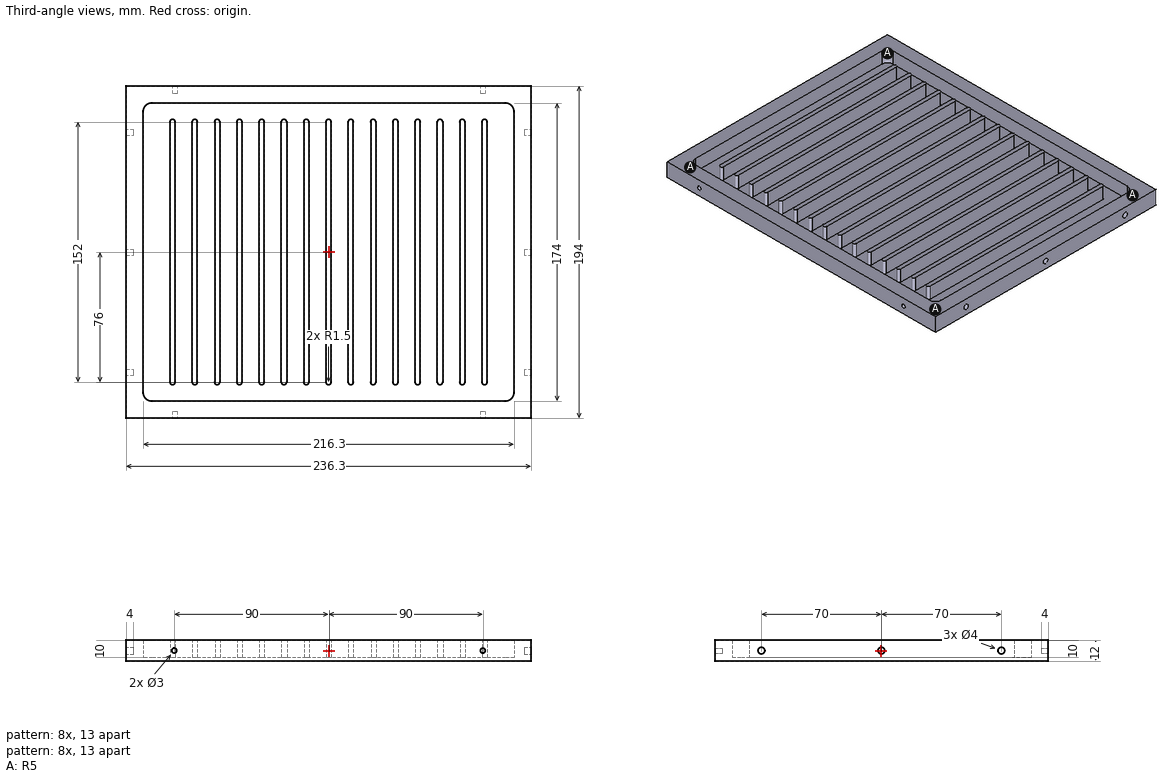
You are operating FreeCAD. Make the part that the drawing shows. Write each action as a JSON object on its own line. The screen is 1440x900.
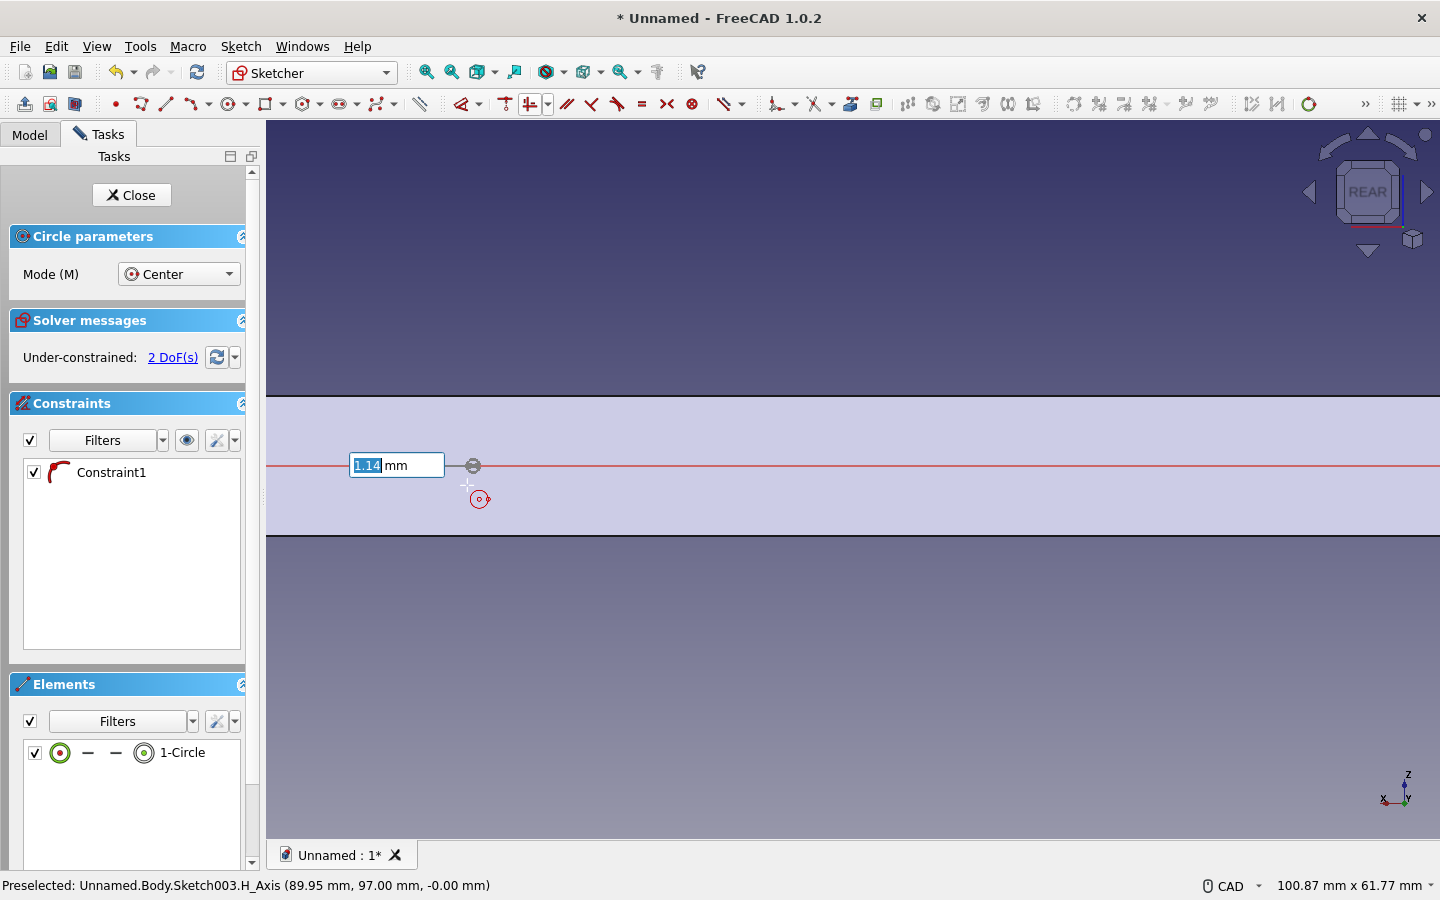
{"action": "left_click", "coordinate": [467, 482]}
{"action": "key", "text": "Escape"}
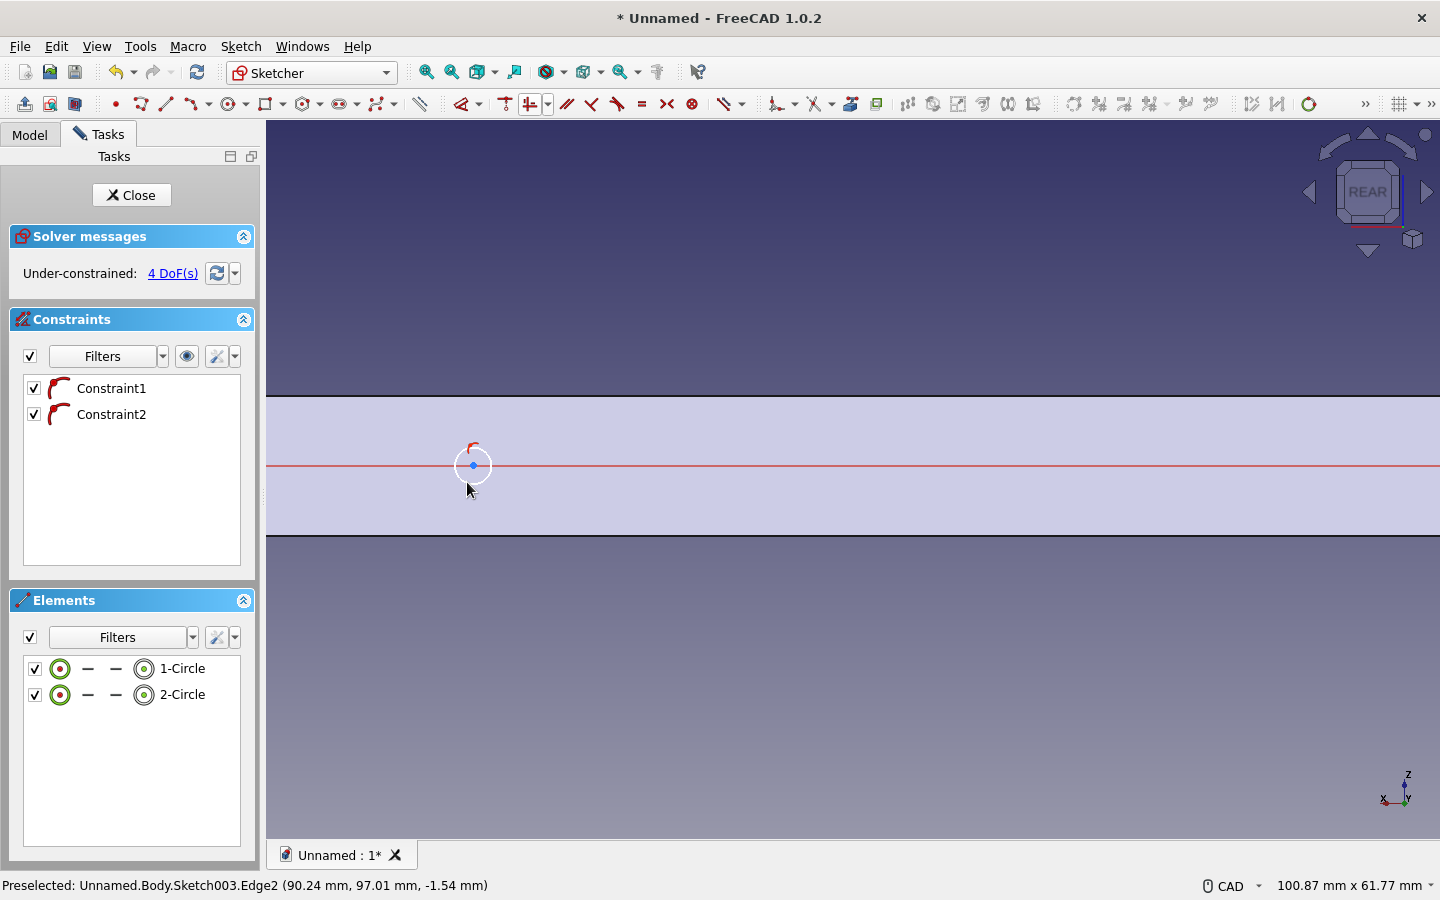
{"action": "scroll", "coordinate": [467, 485], "scroll_direction": "down", "scroll_amount": 6}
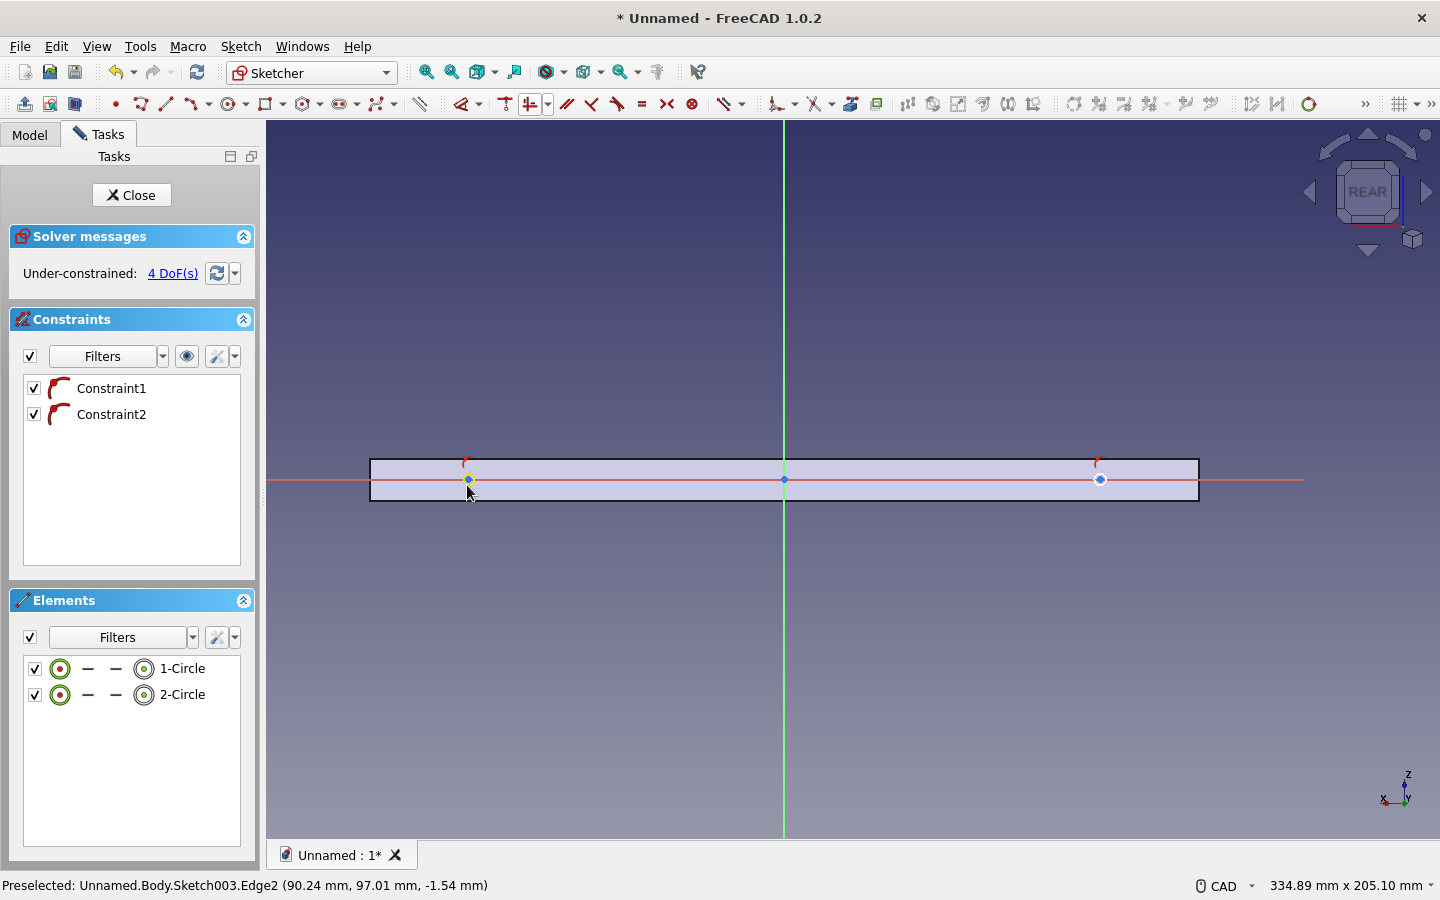
{"action": "scroll", "coordinate": [1104, 476], "scroll_direction": "up", "scroll_amount": 7}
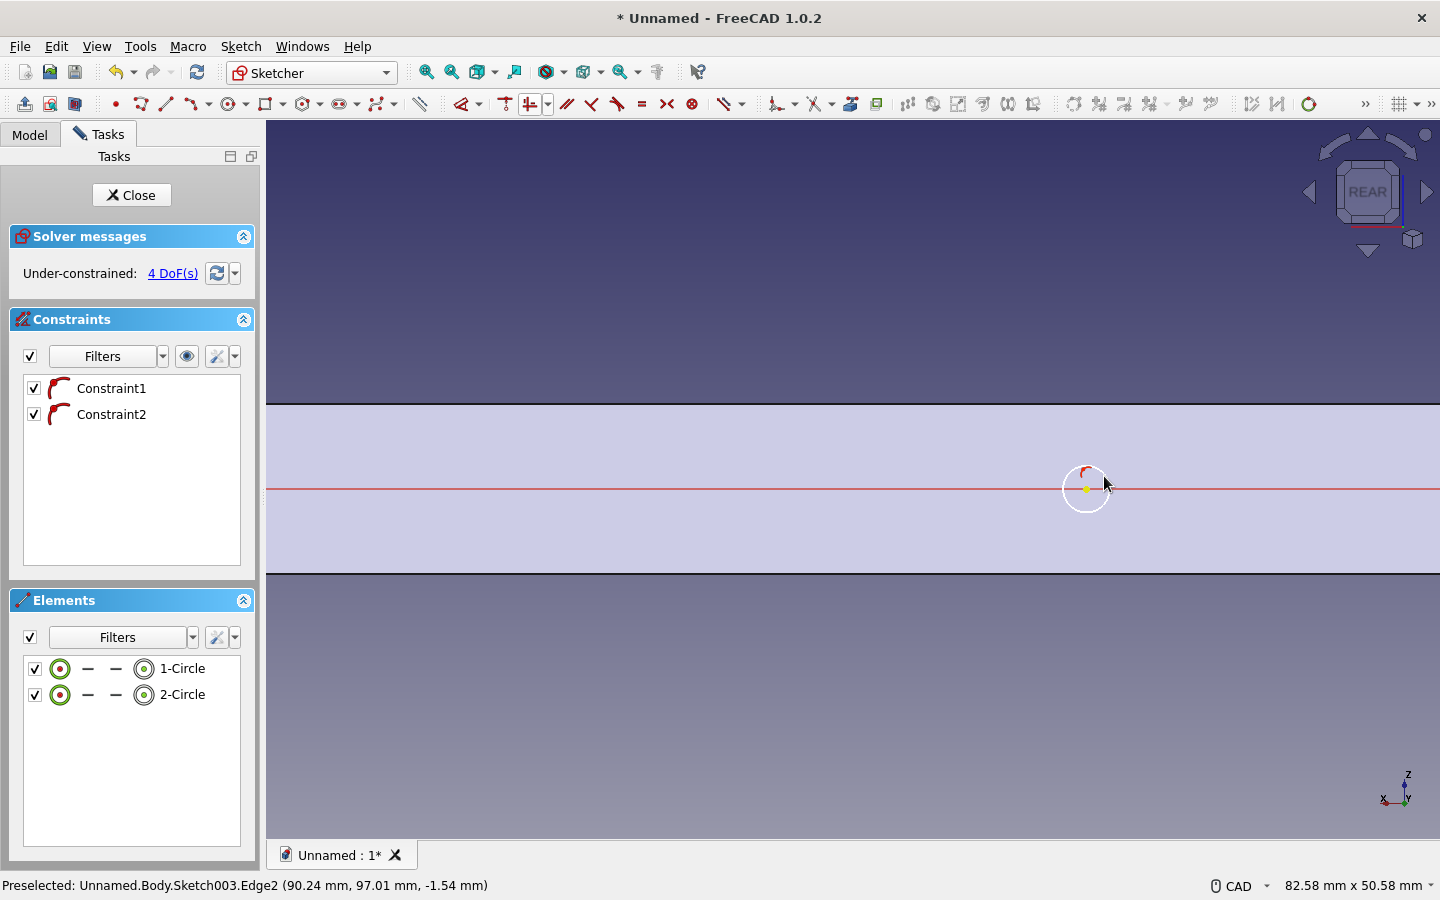
{"action": "left_click", "coordinate": [1103, 473]}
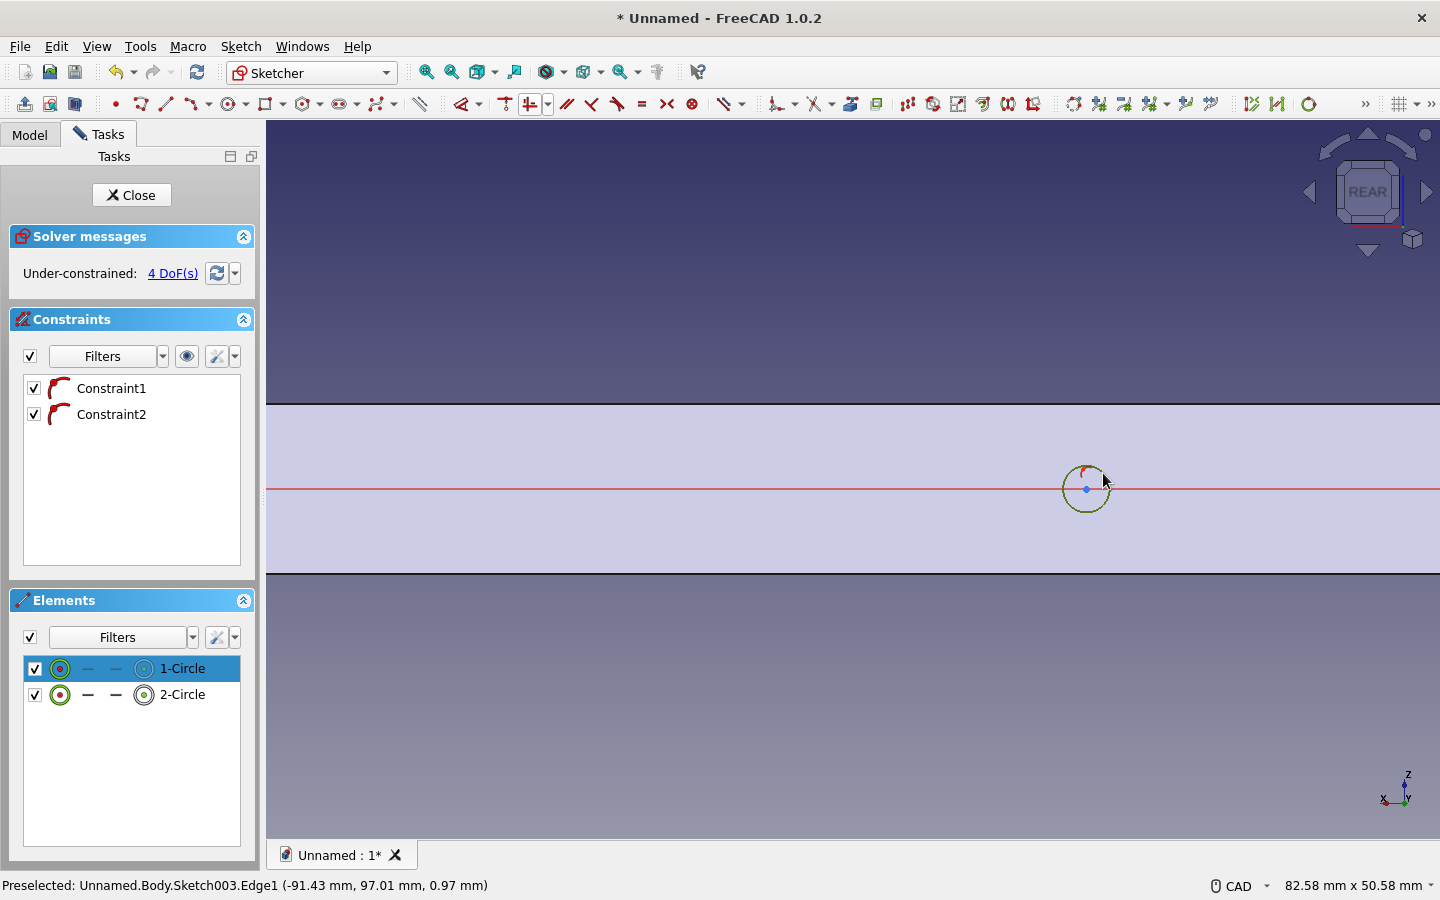
{"action": "scroll", "coordinate": [1105, 476], "scroll_direction": "down", "scroll_amount": 7}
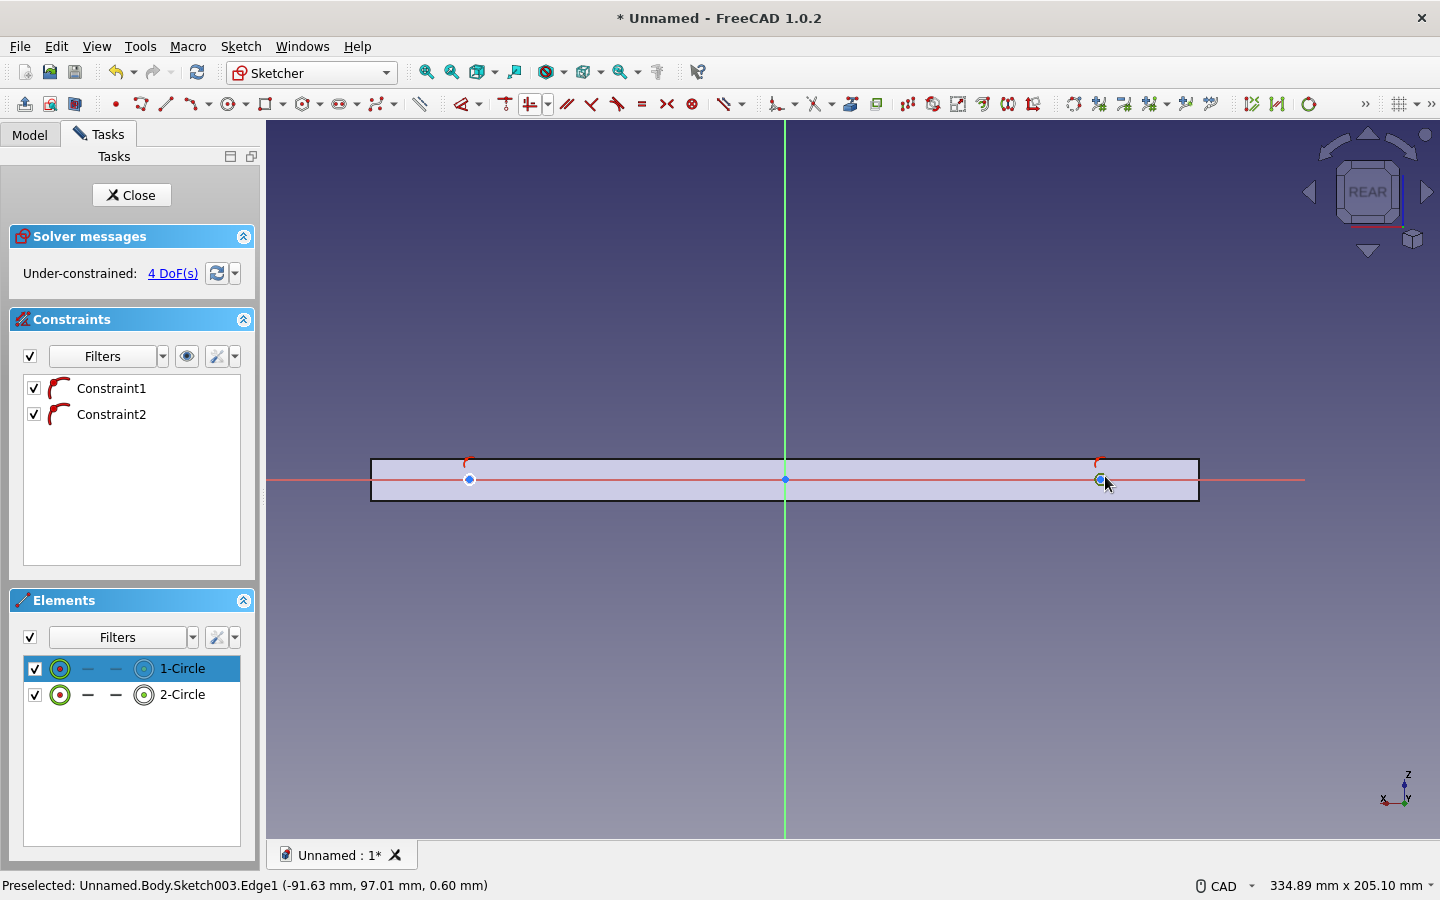
{"action": "scroll", "coordinate": [474, 476], "scroll_direction": "up", "scroll_amount": 7}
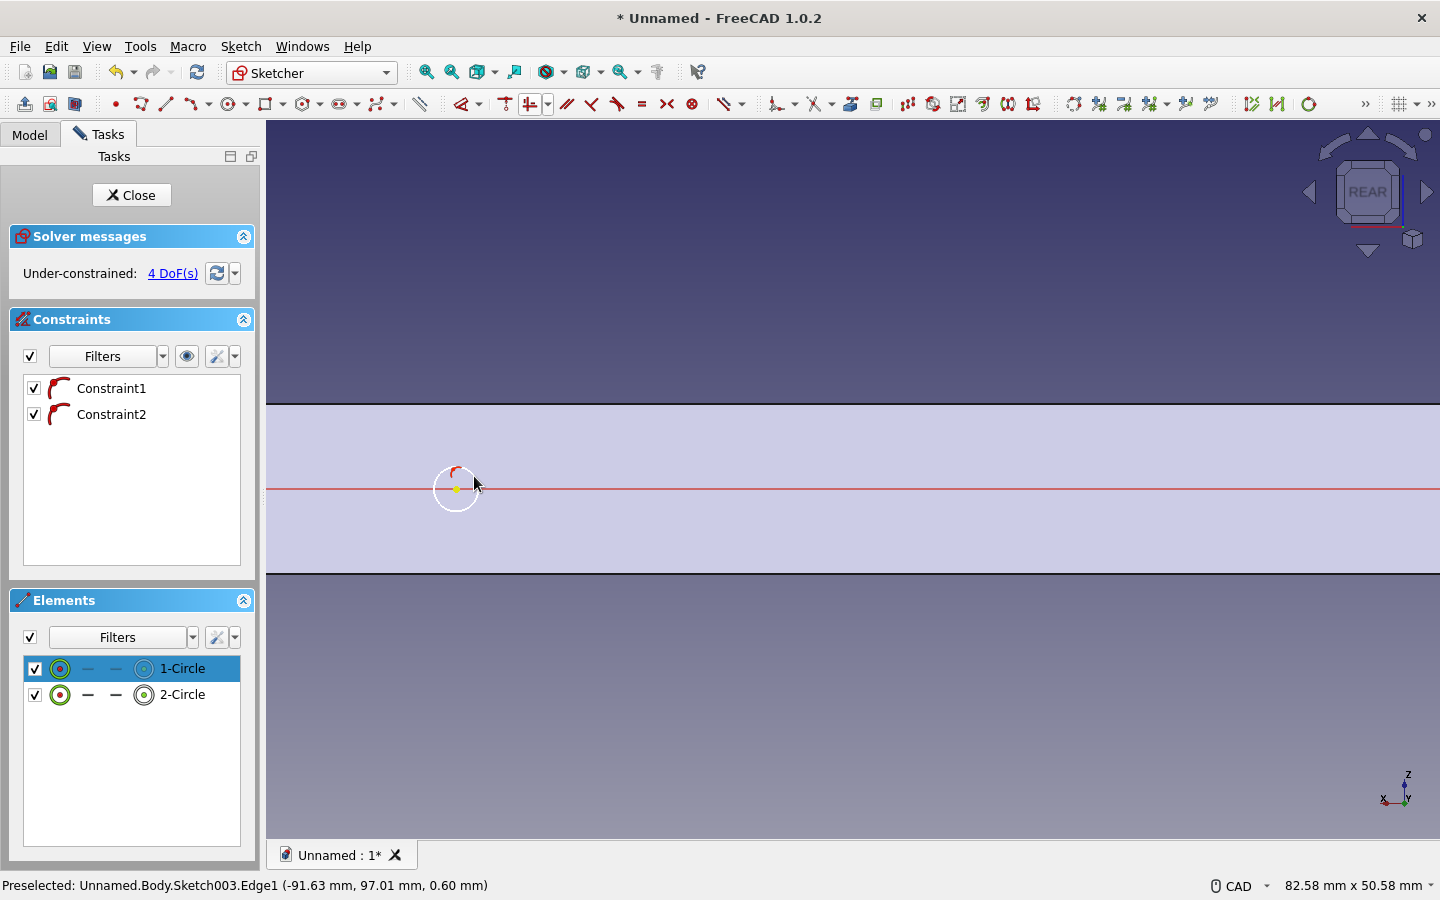
{"action": "left_click", "coordinate": [472, 473]}